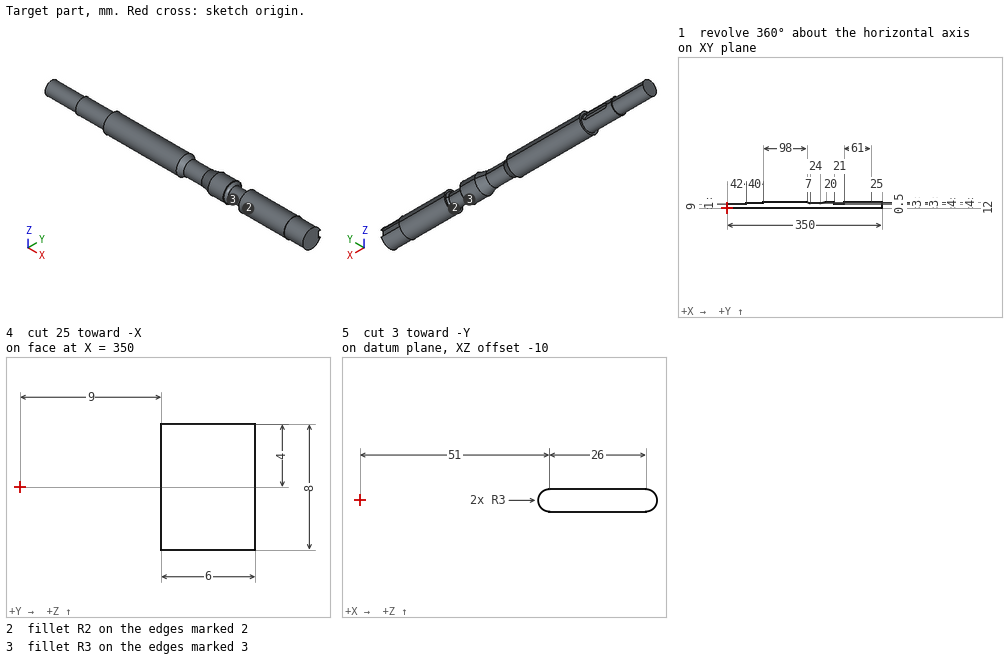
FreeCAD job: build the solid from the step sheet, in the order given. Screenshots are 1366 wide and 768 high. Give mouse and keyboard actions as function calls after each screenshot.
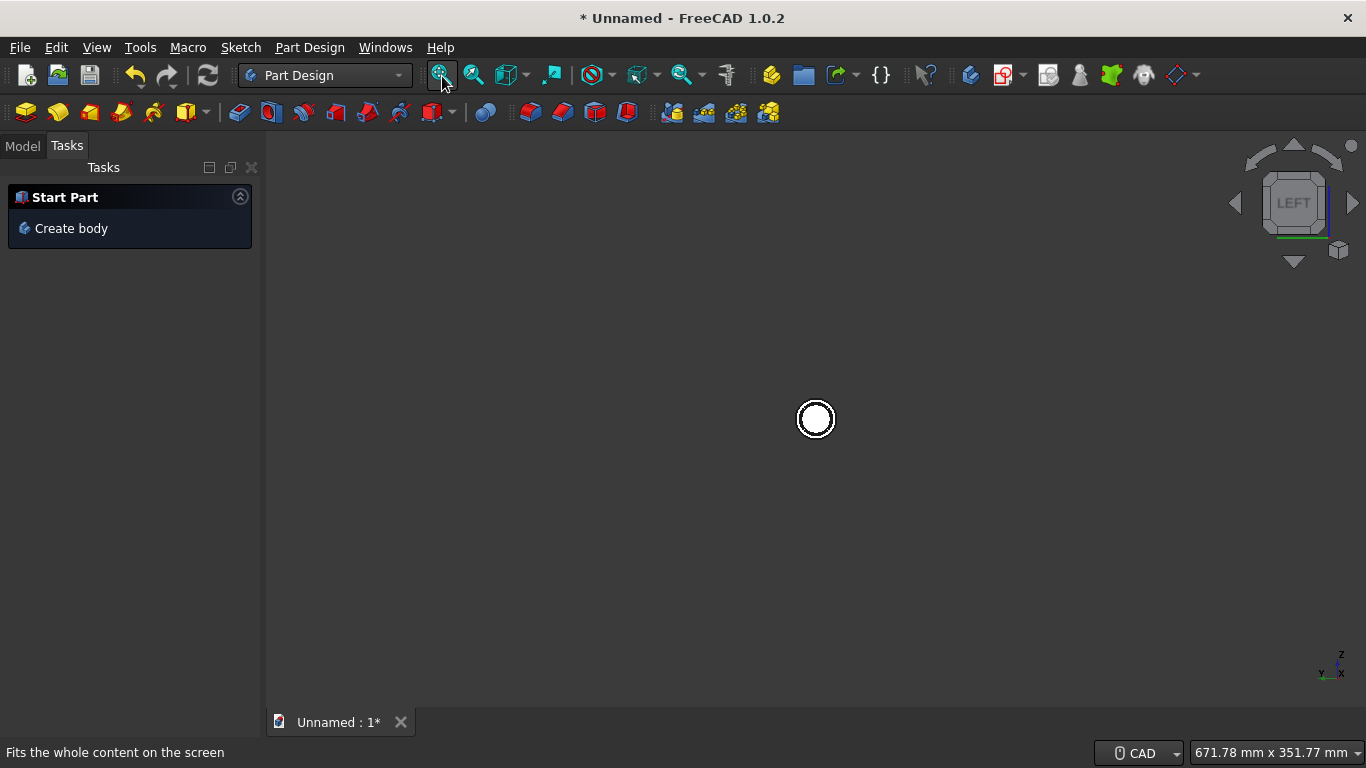
key(v)
key(3)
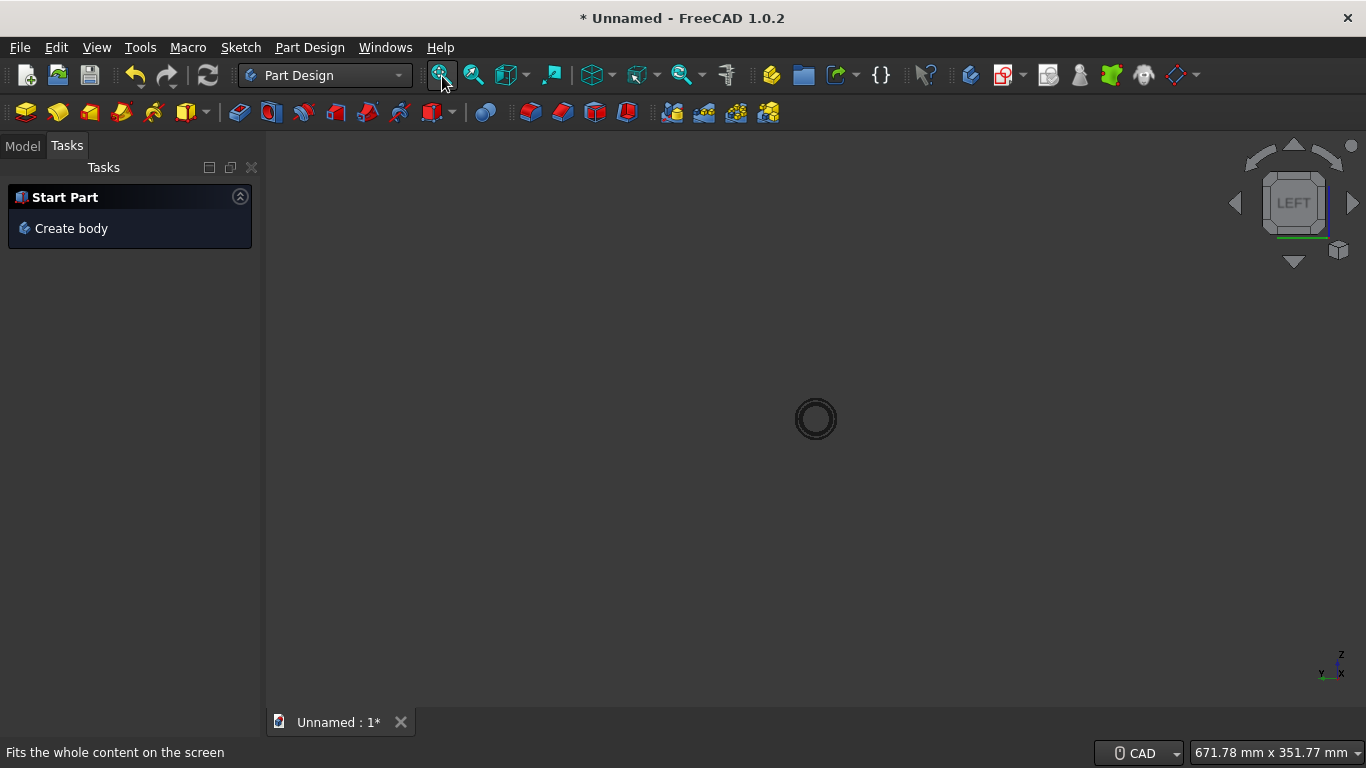
key(0)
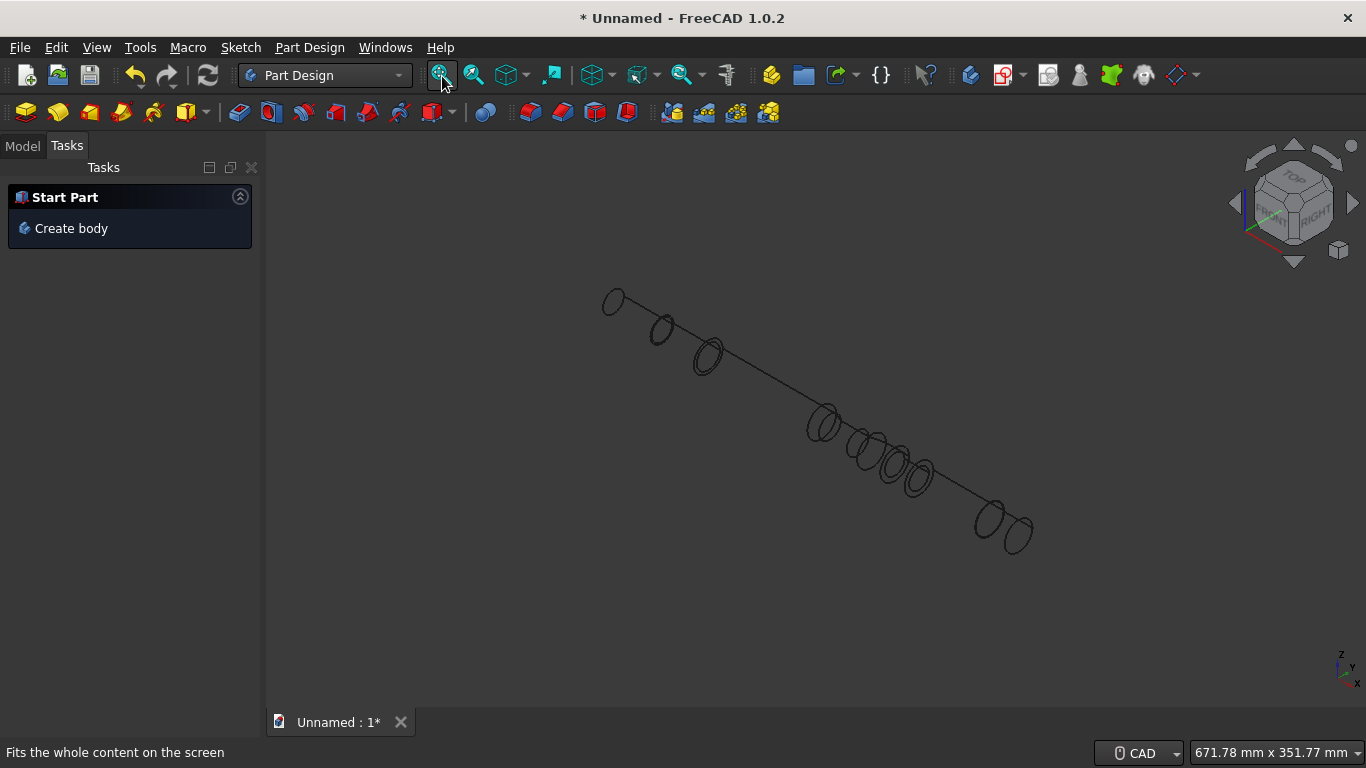
click(916, 490)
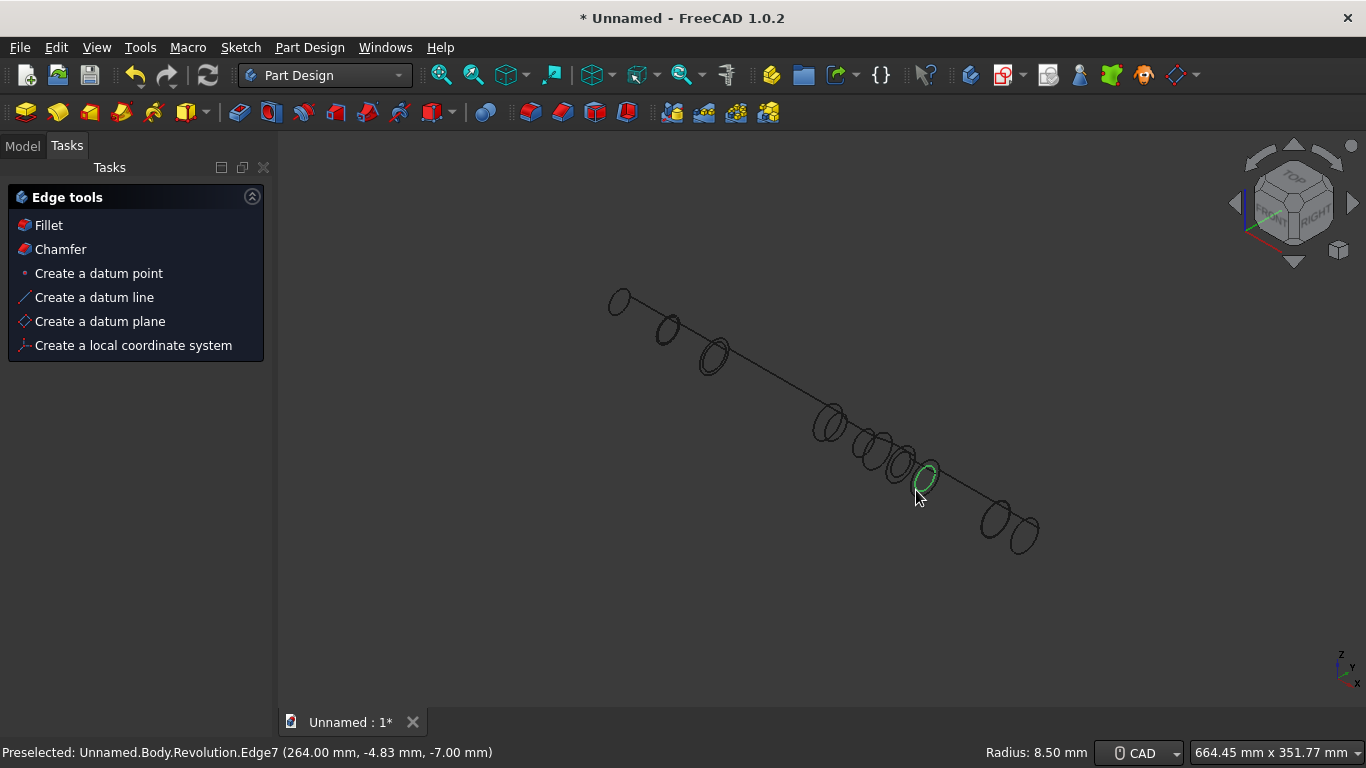
key(v)
key(1)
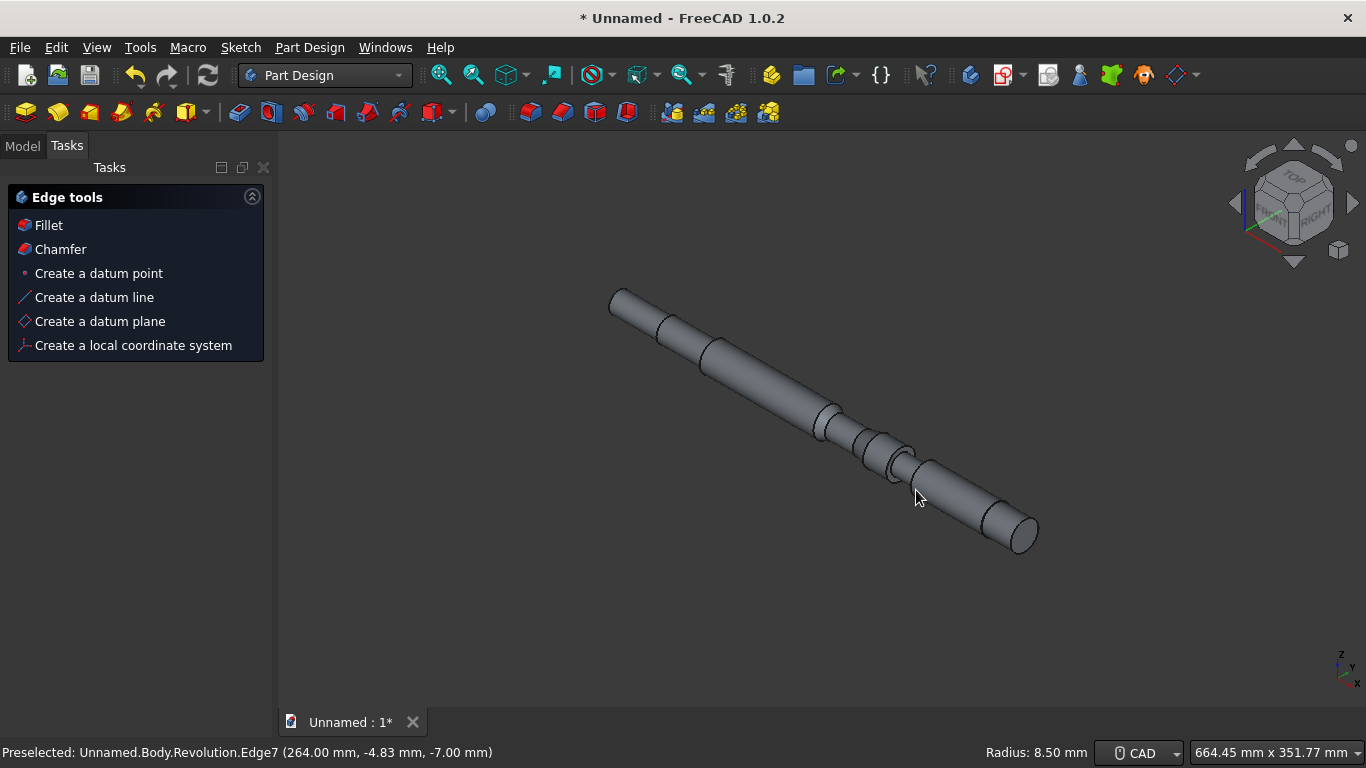
click(532, 112)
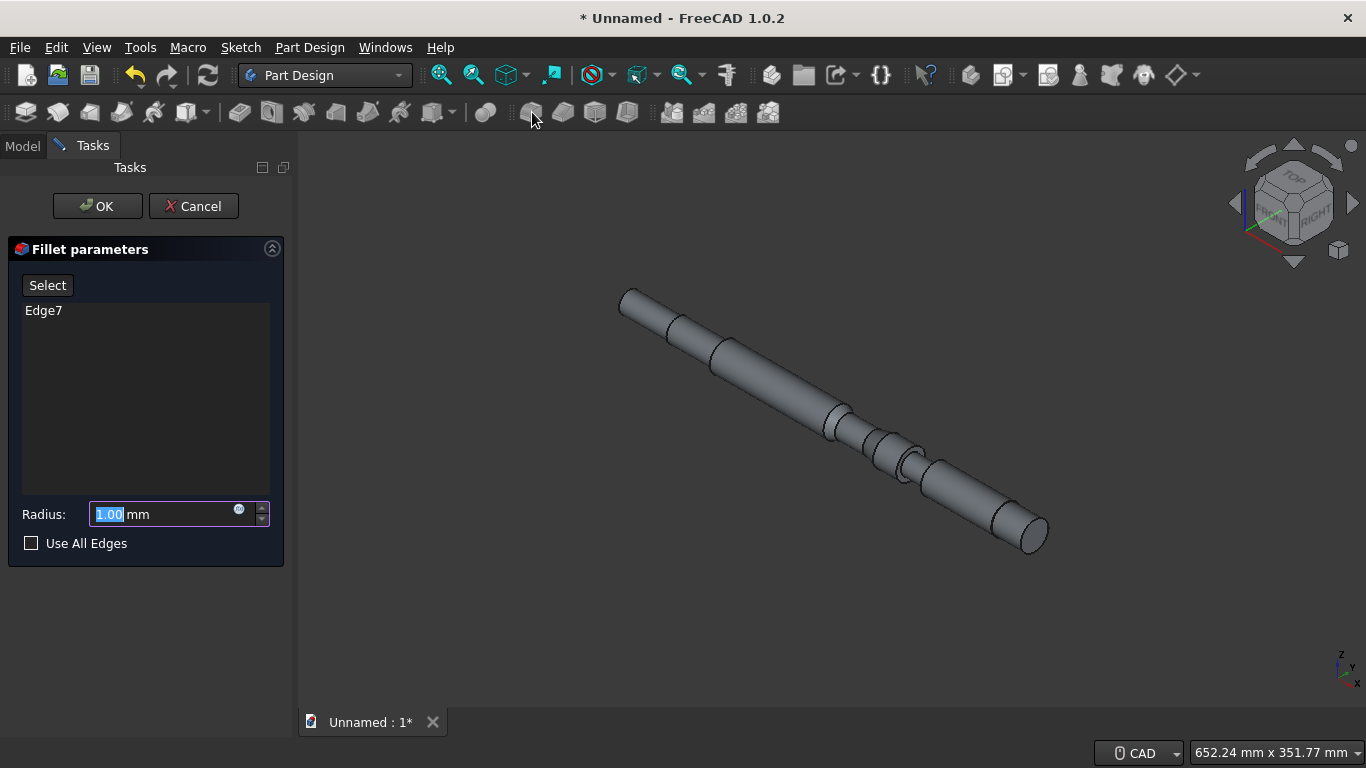
text(2)
key(Tab)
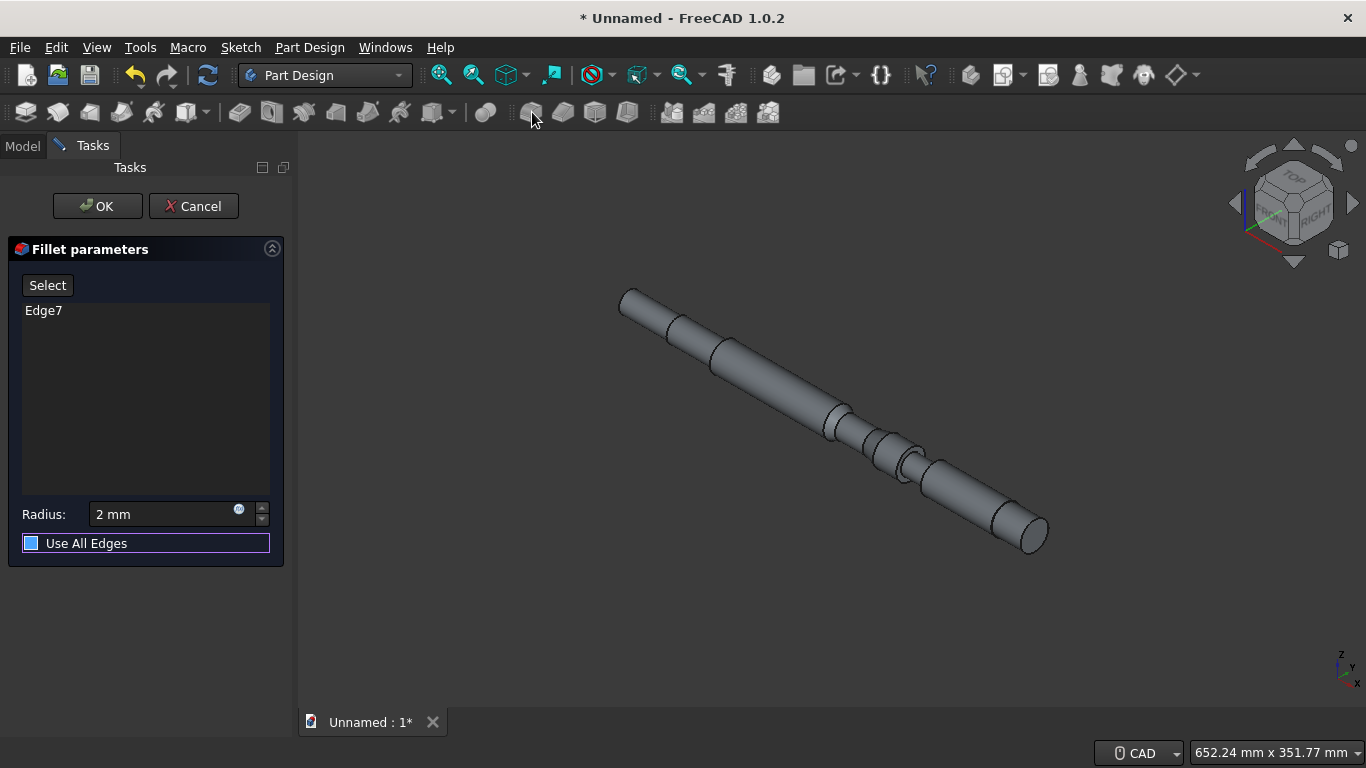
click(98, 206)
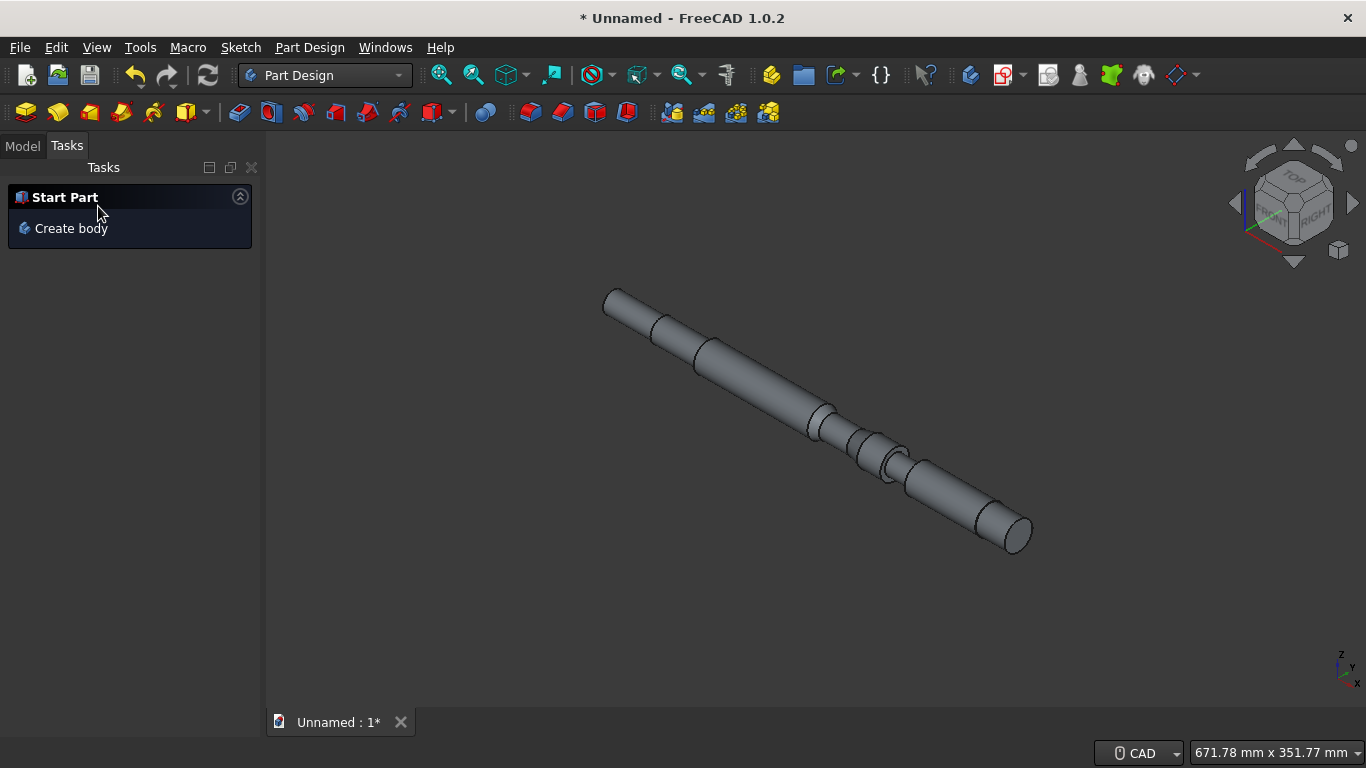
key(2)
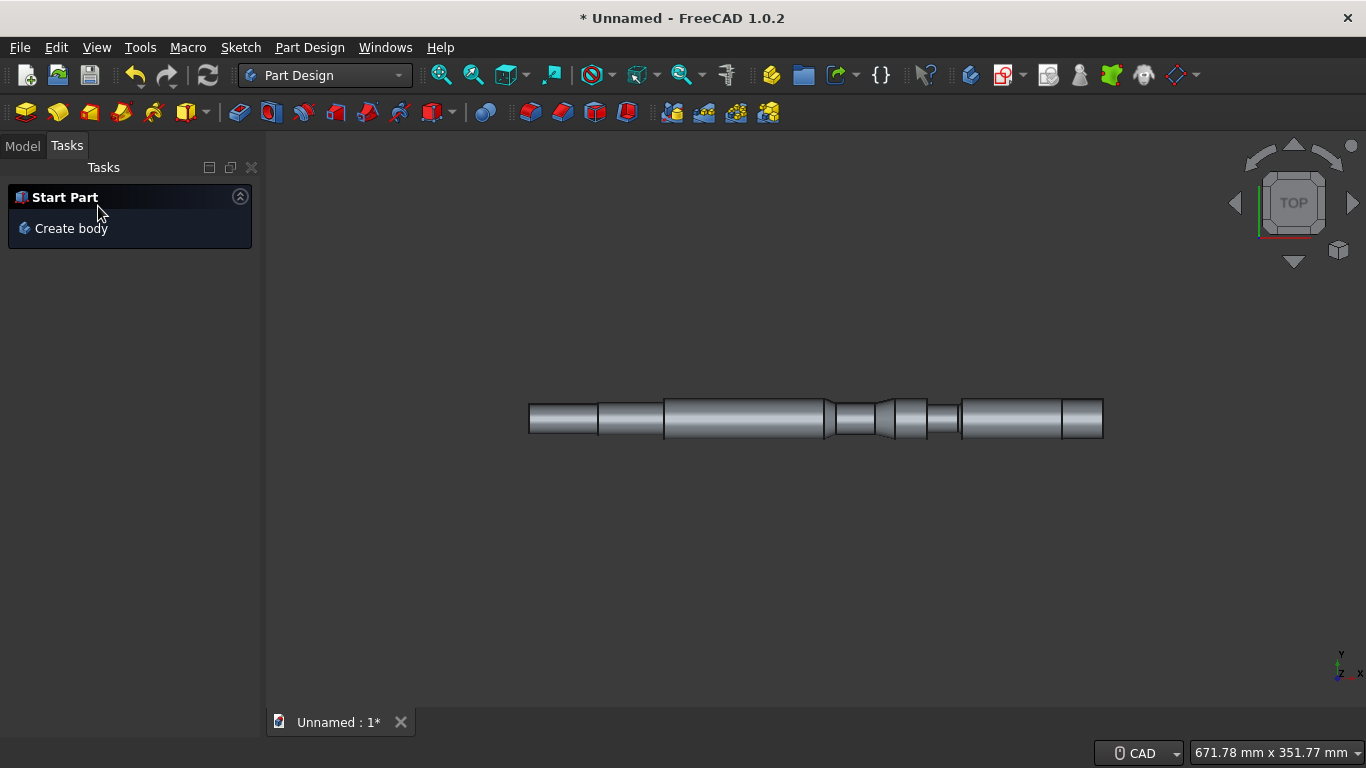
key(0)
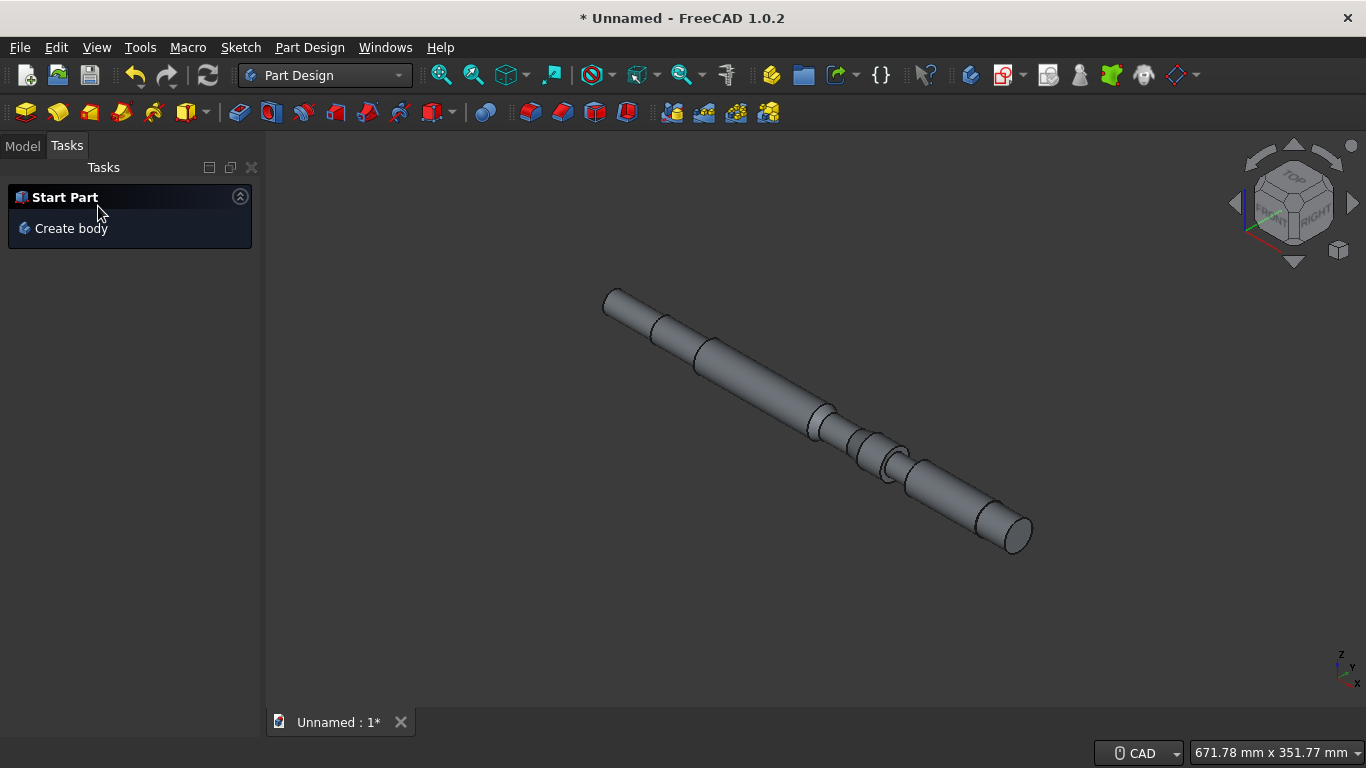
key(1)